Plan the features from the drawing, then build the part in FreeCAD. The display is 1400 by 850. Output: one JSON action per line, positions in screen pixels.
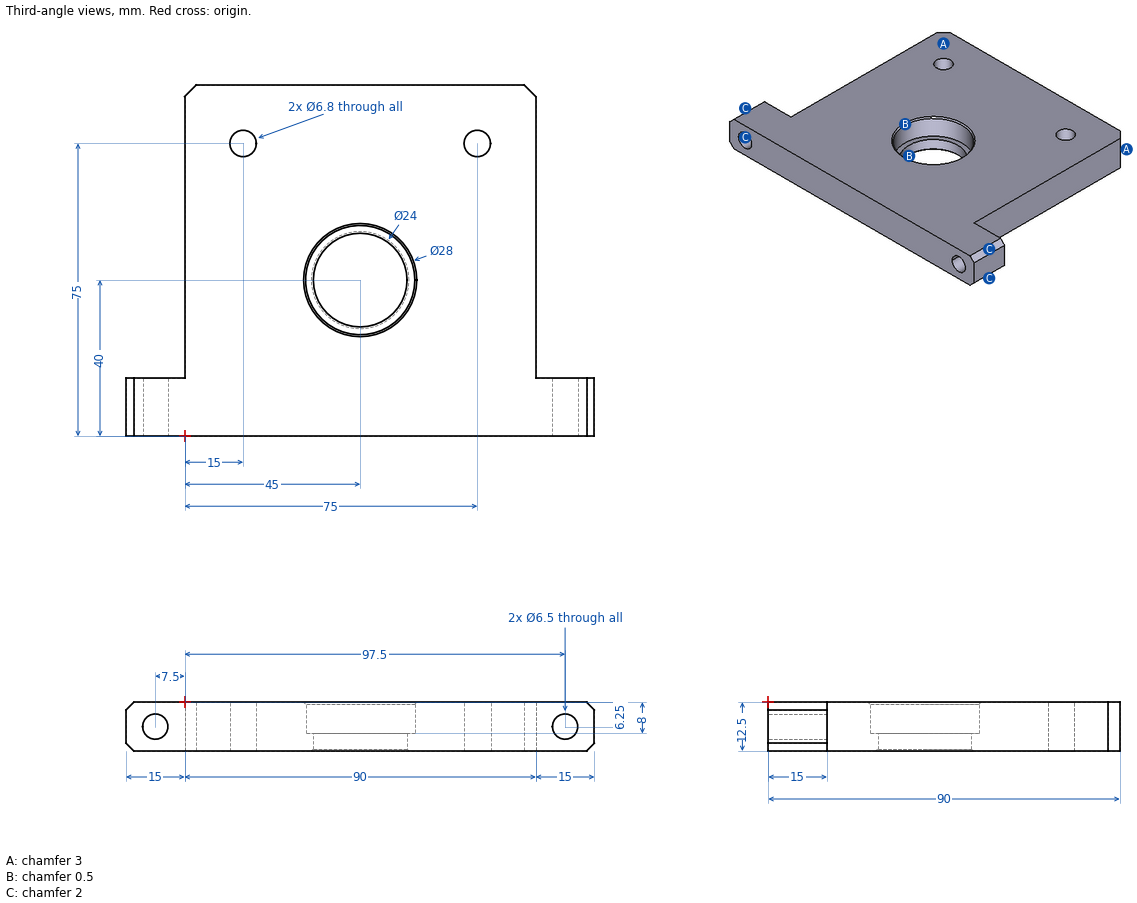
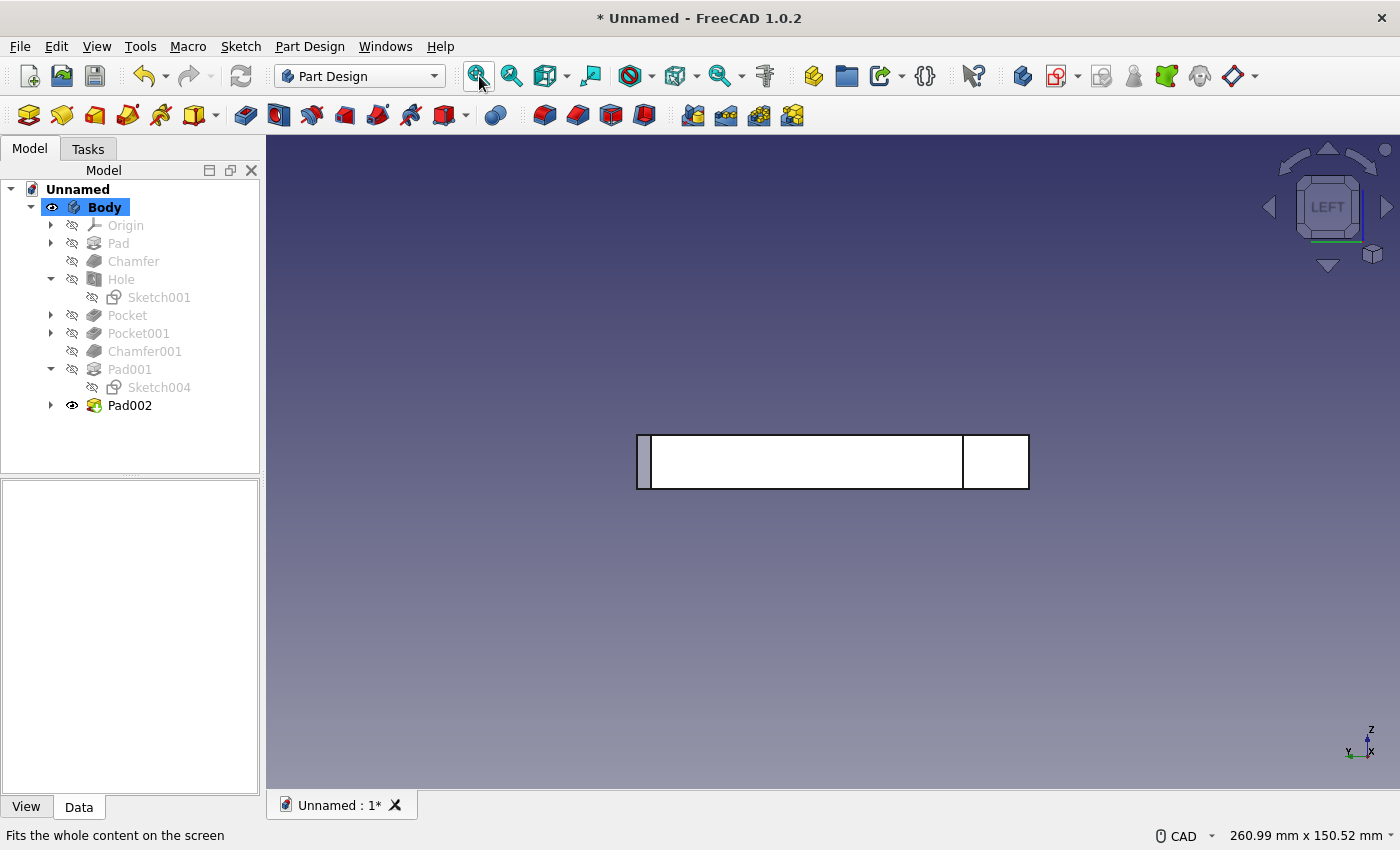
{"action": "left_click", "coordinate": [996, 434]}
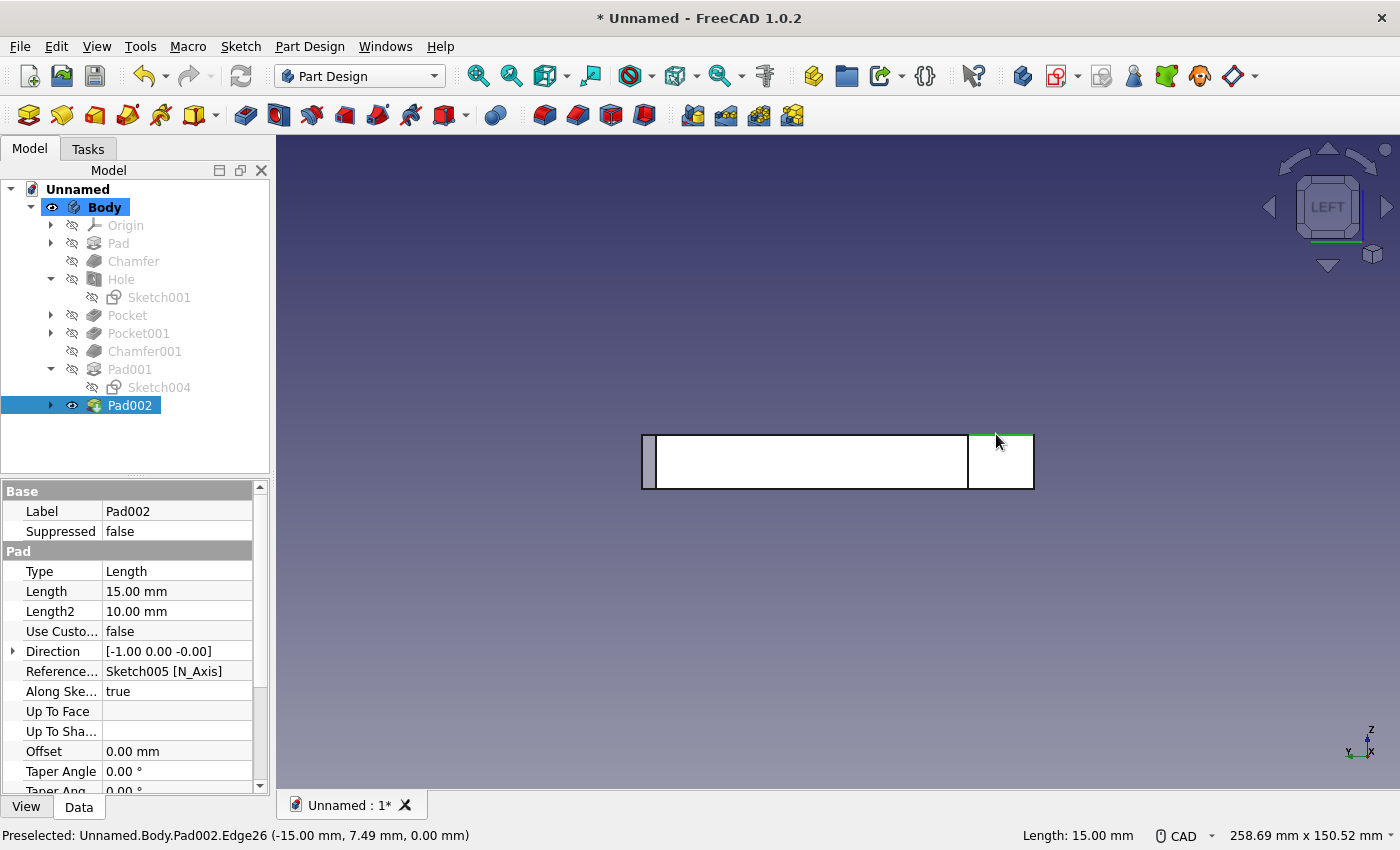
{"action": "left_click", "coordinate": [1001, 488], "text": "ctrl"}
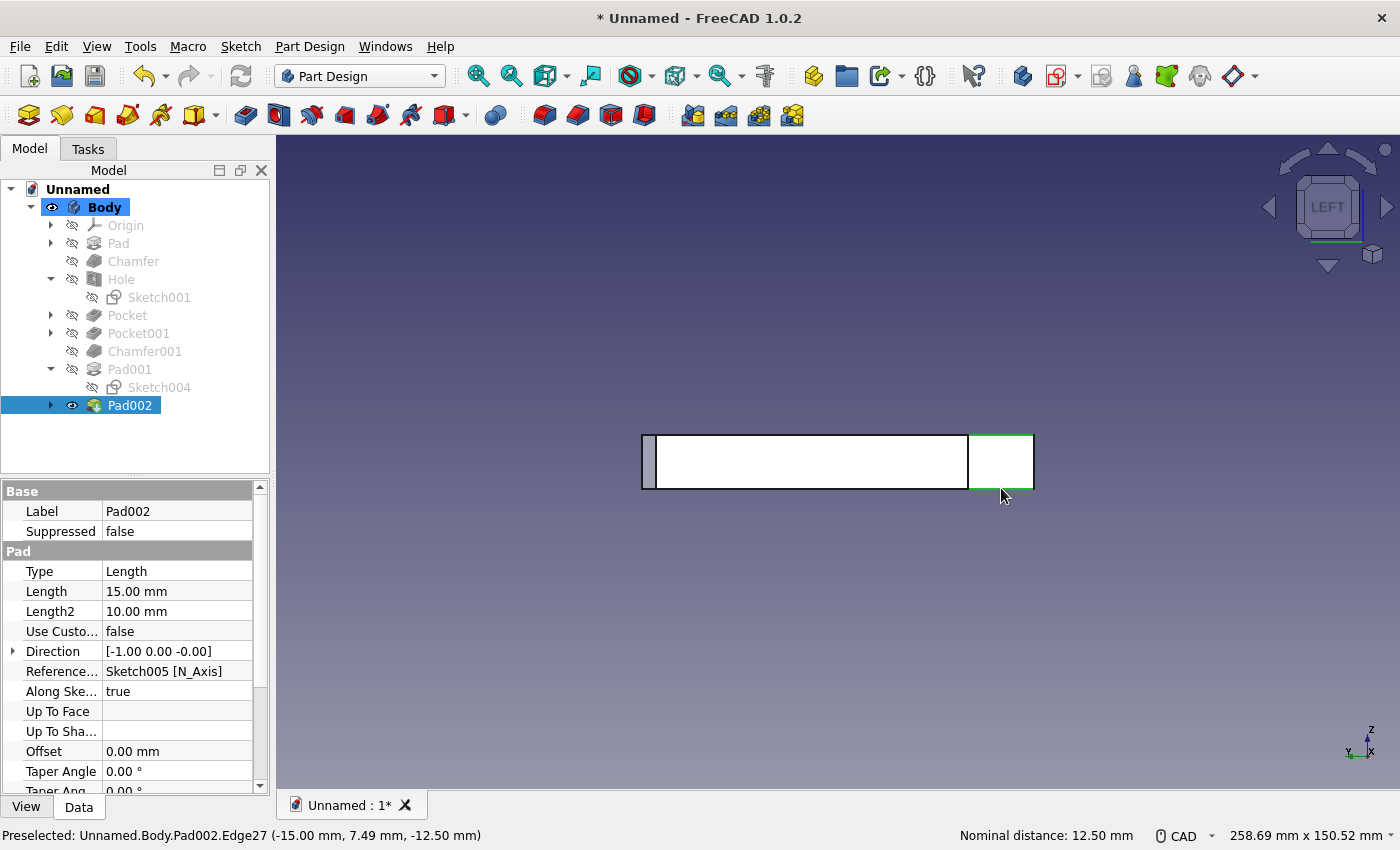
{"action": "key", "text": "0"}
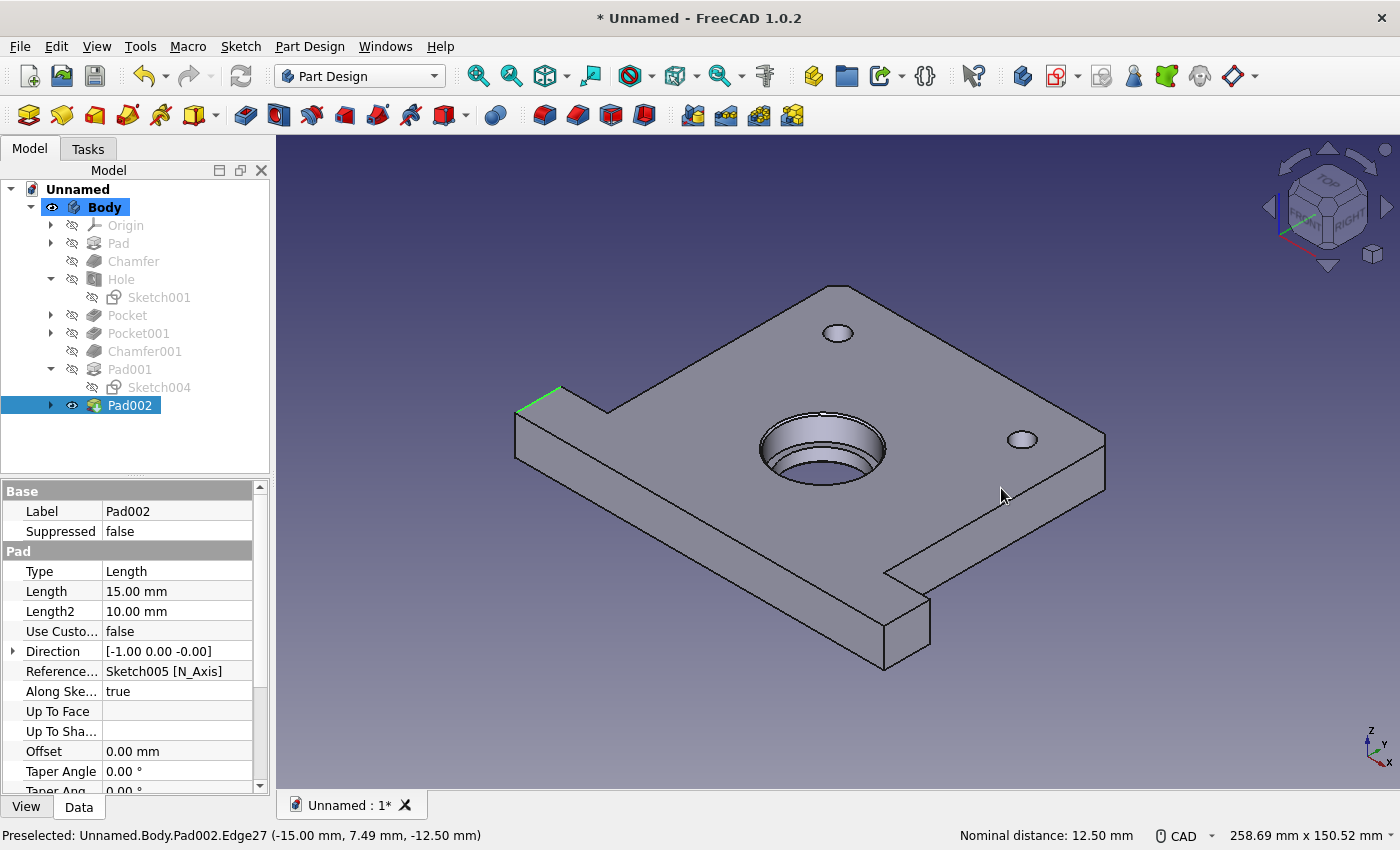
{"action": "left_click", "coordinate": [907, 612], "text": "ctrl"}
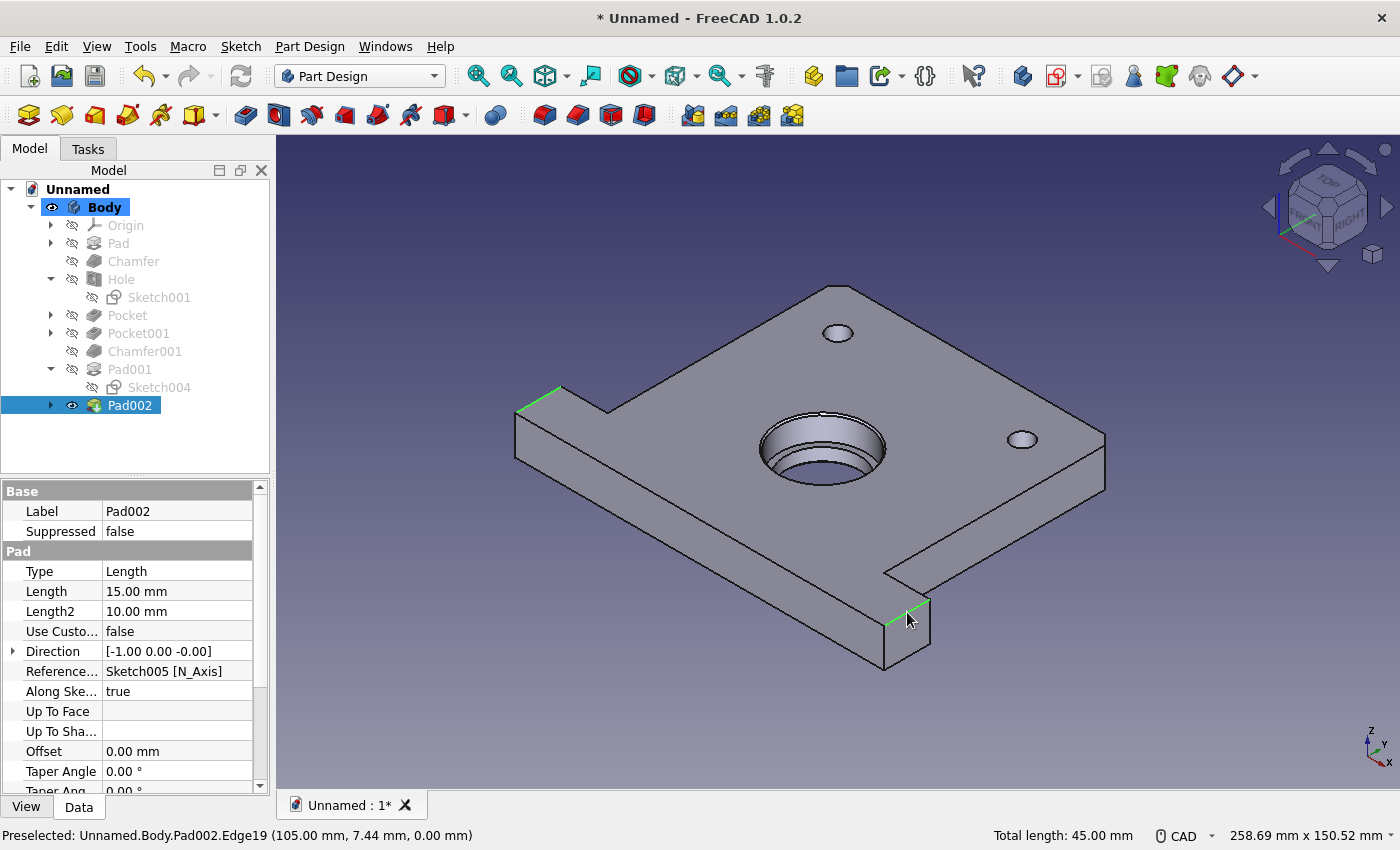
{"action": "key", "text": "2"}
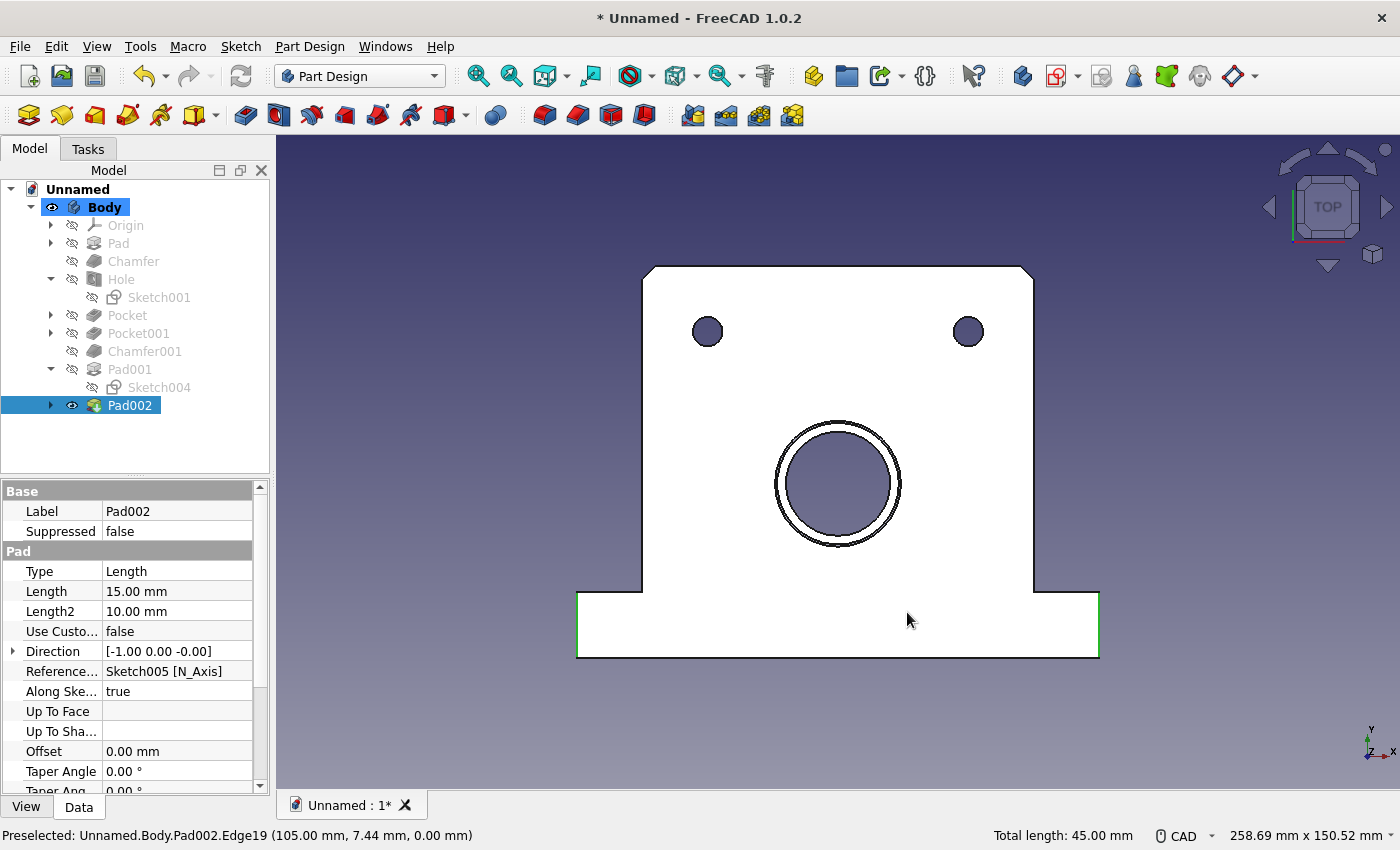
{"action": "key", "text": "1"}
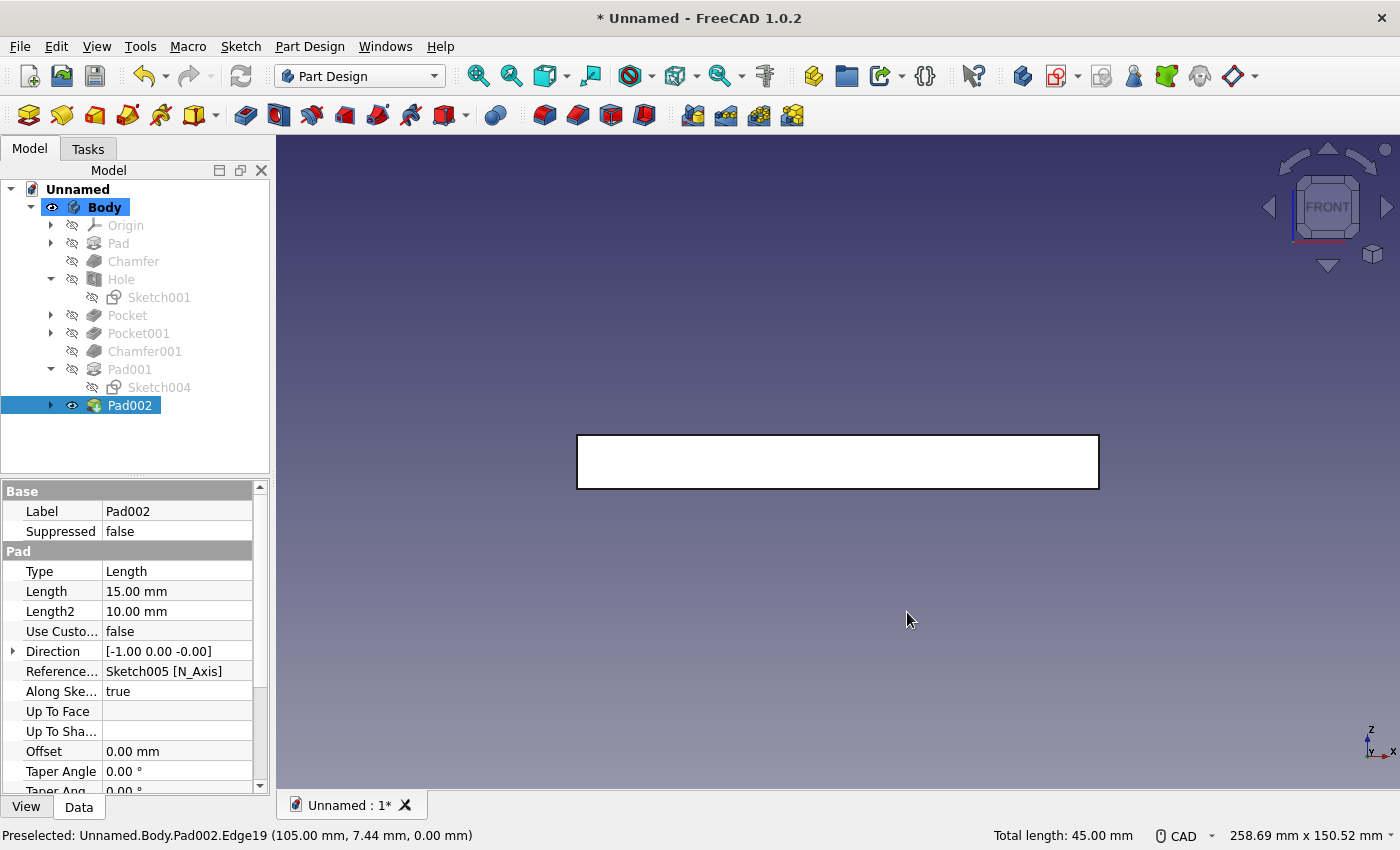
{"action": "key", "text": "3"}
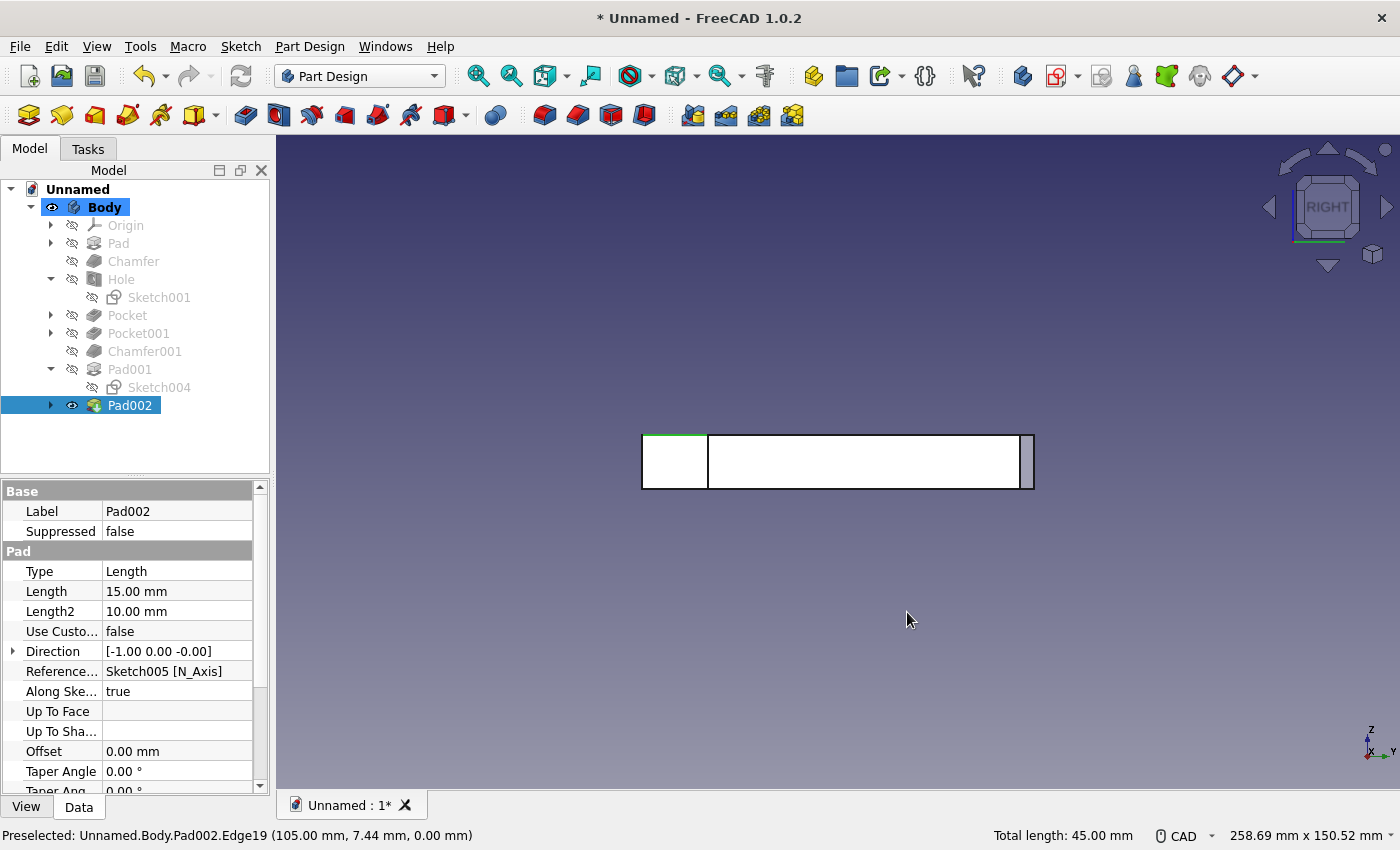
{"action": "left_click", "coordinate": [479, 76]}